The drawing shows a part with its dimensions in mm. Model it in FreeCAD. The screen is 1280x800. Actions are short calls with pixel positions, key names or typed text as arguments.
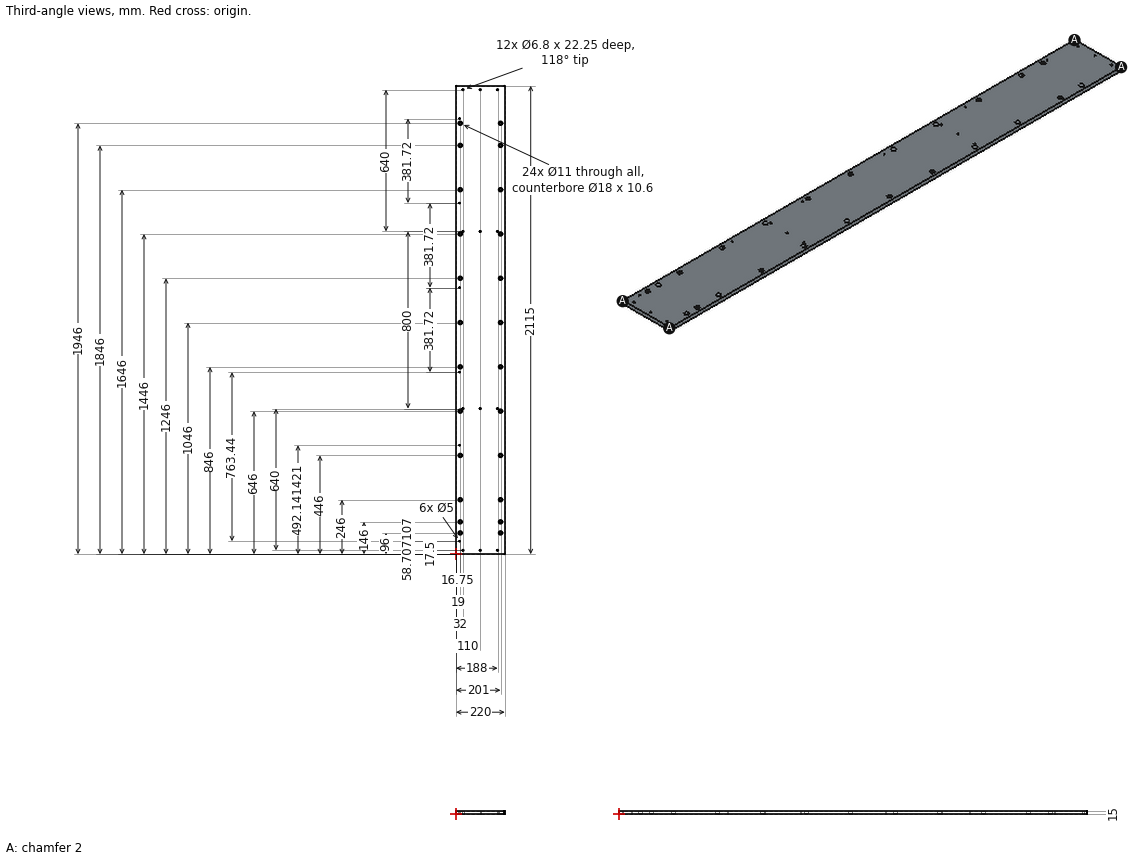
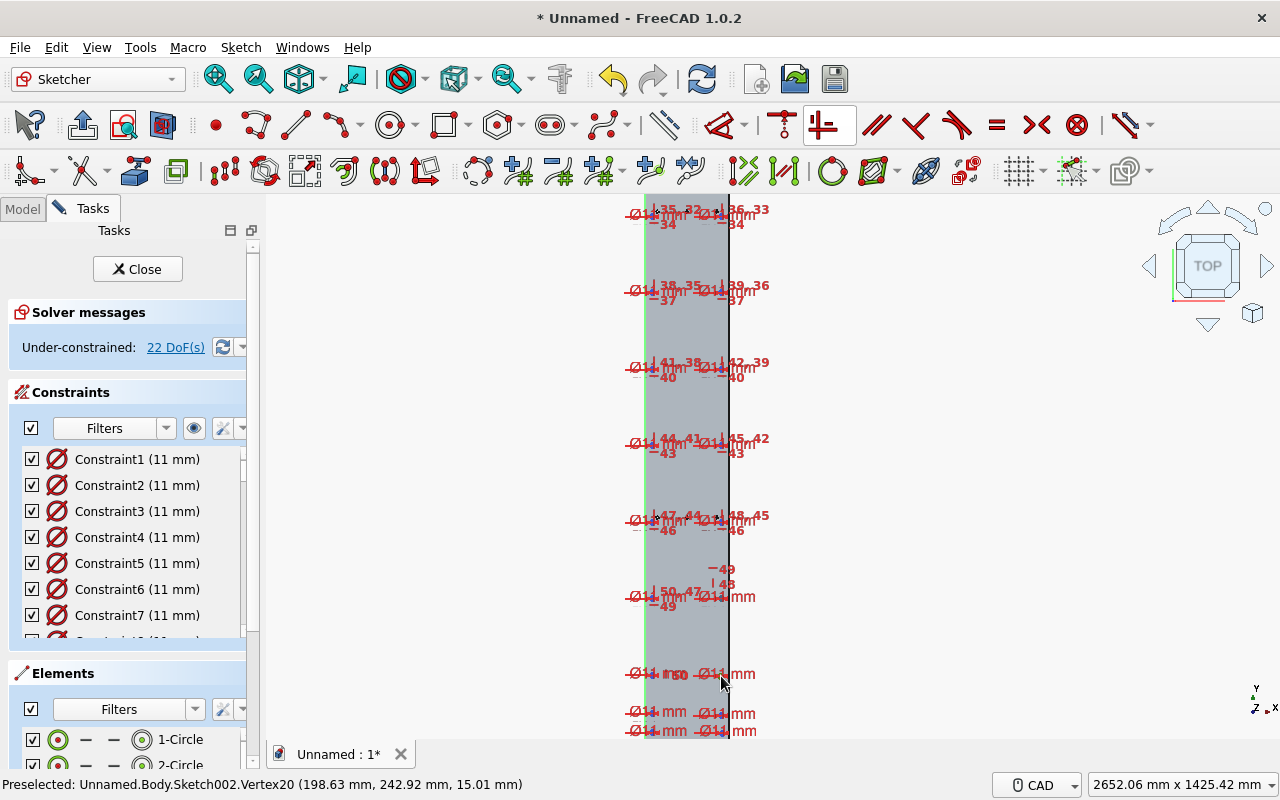
click(850, 126)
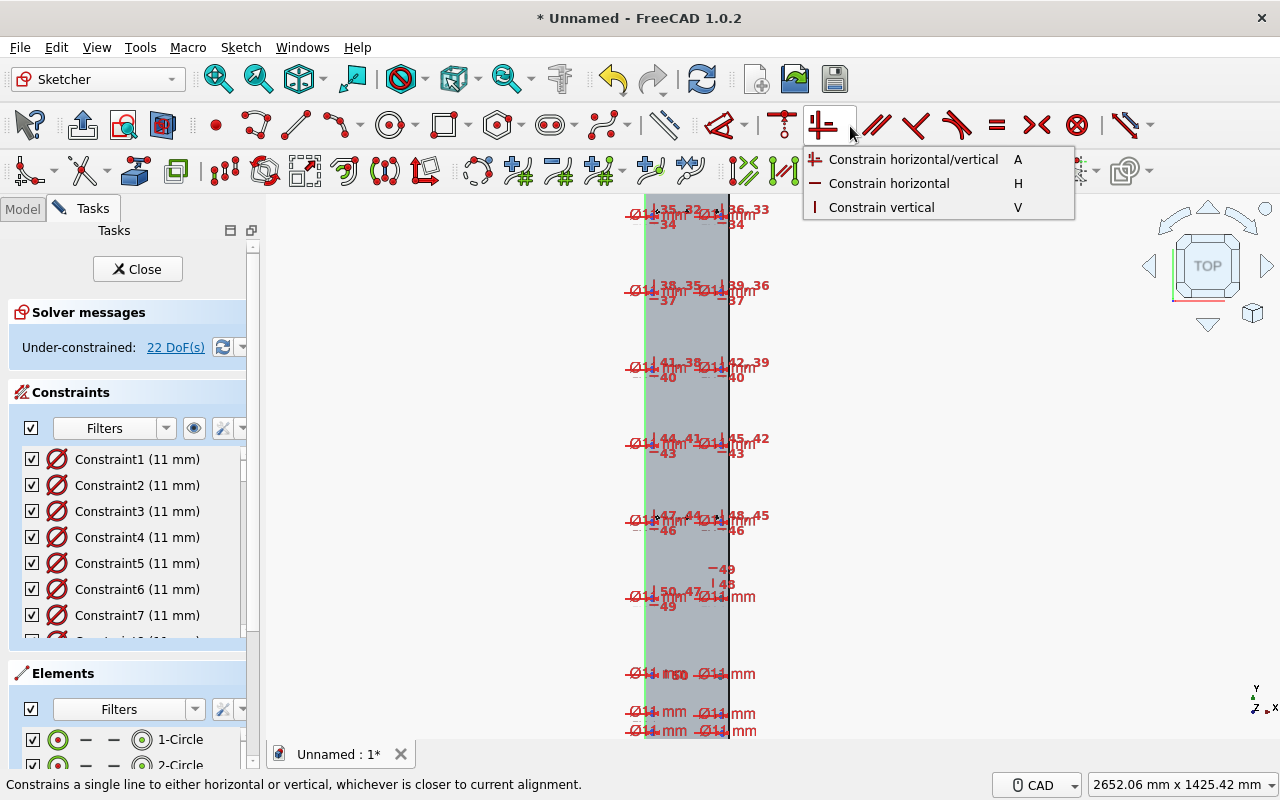
click(939, 207)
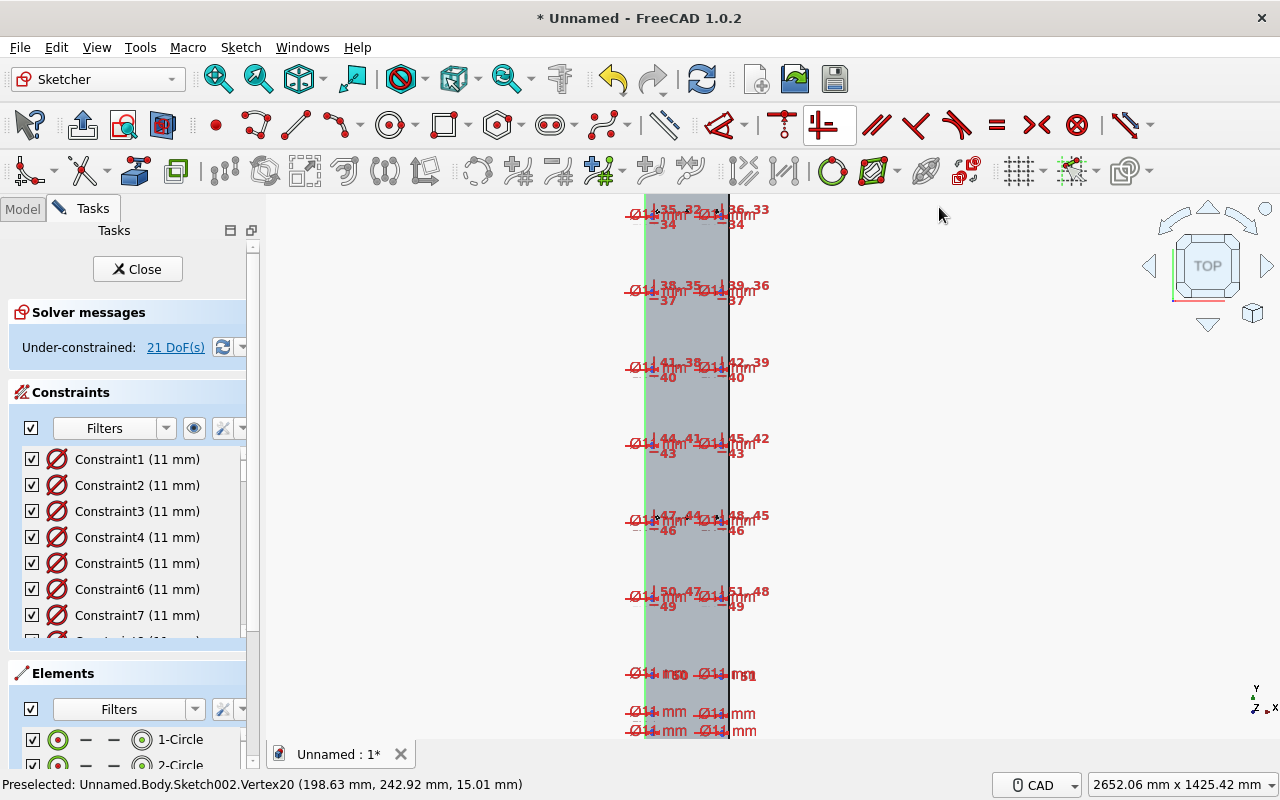
click(652, 675)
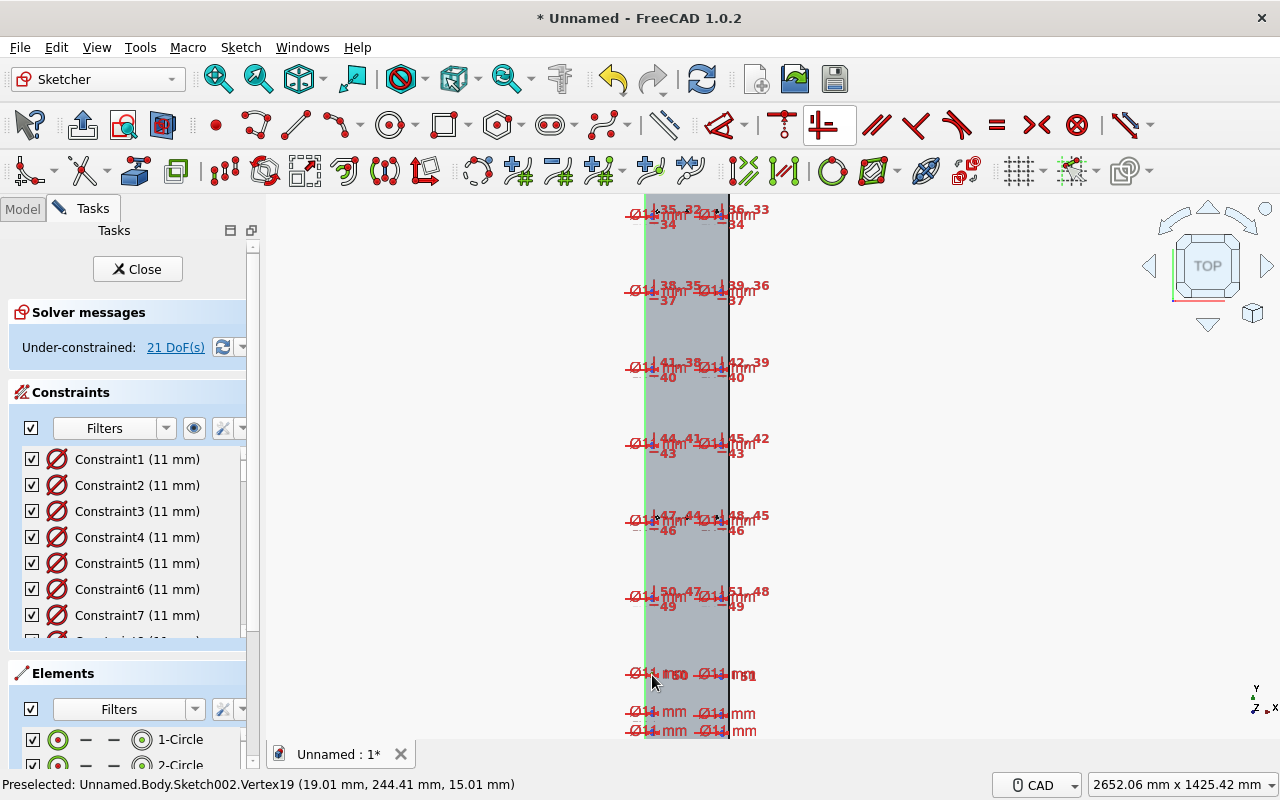
click(721, 676)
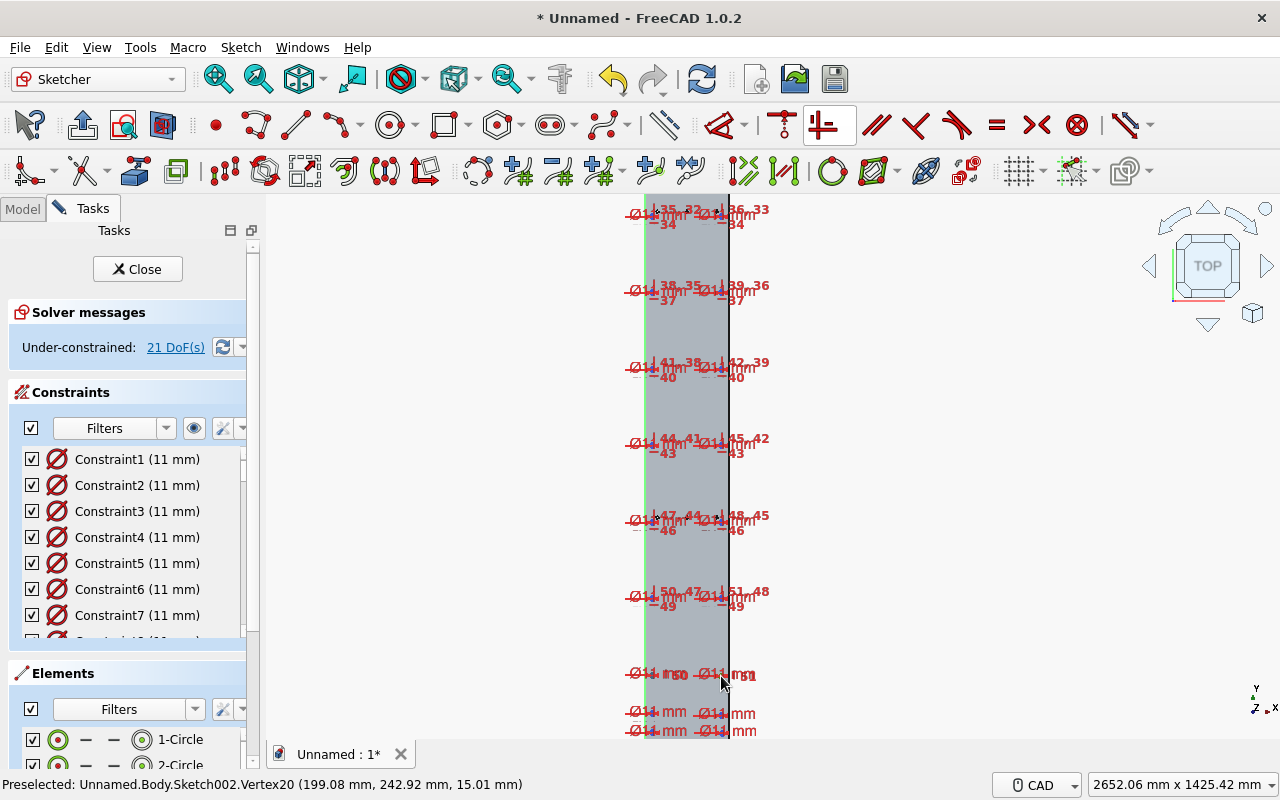
click(850, 126)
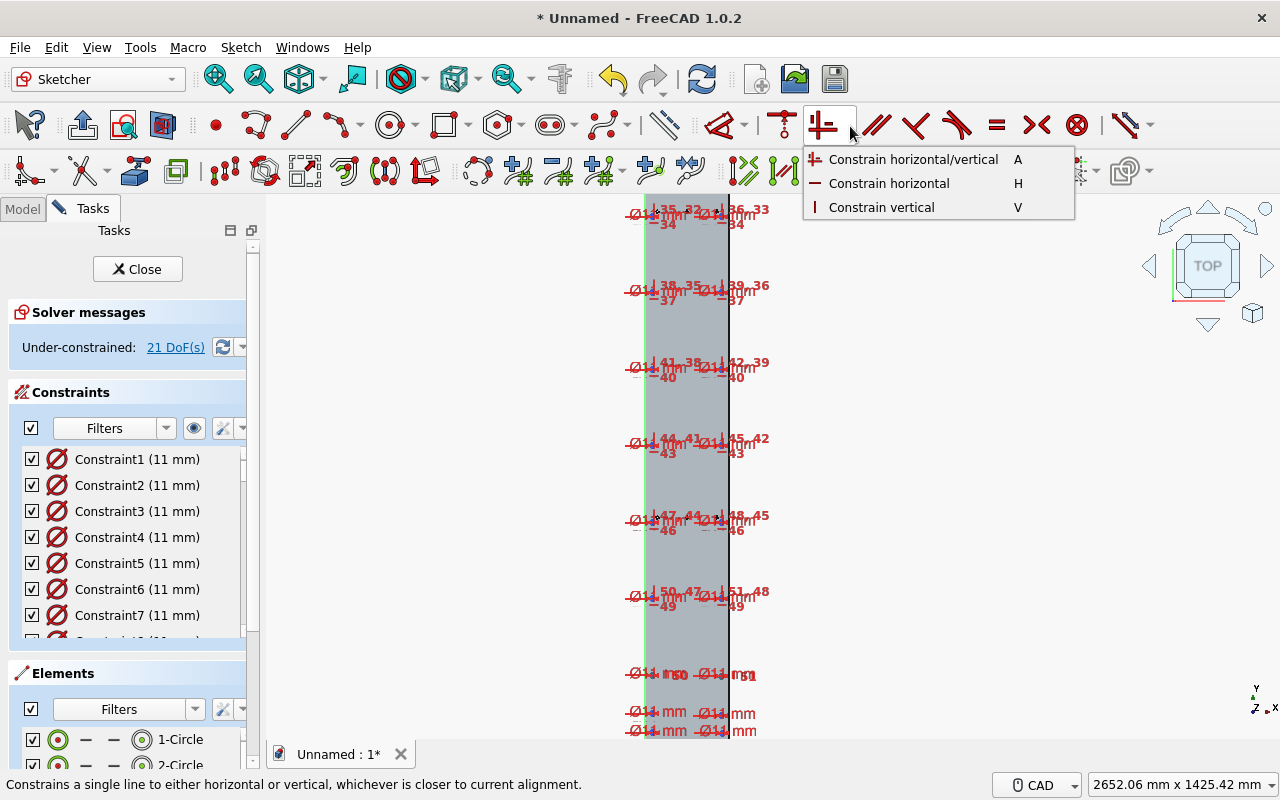
click(939, 183)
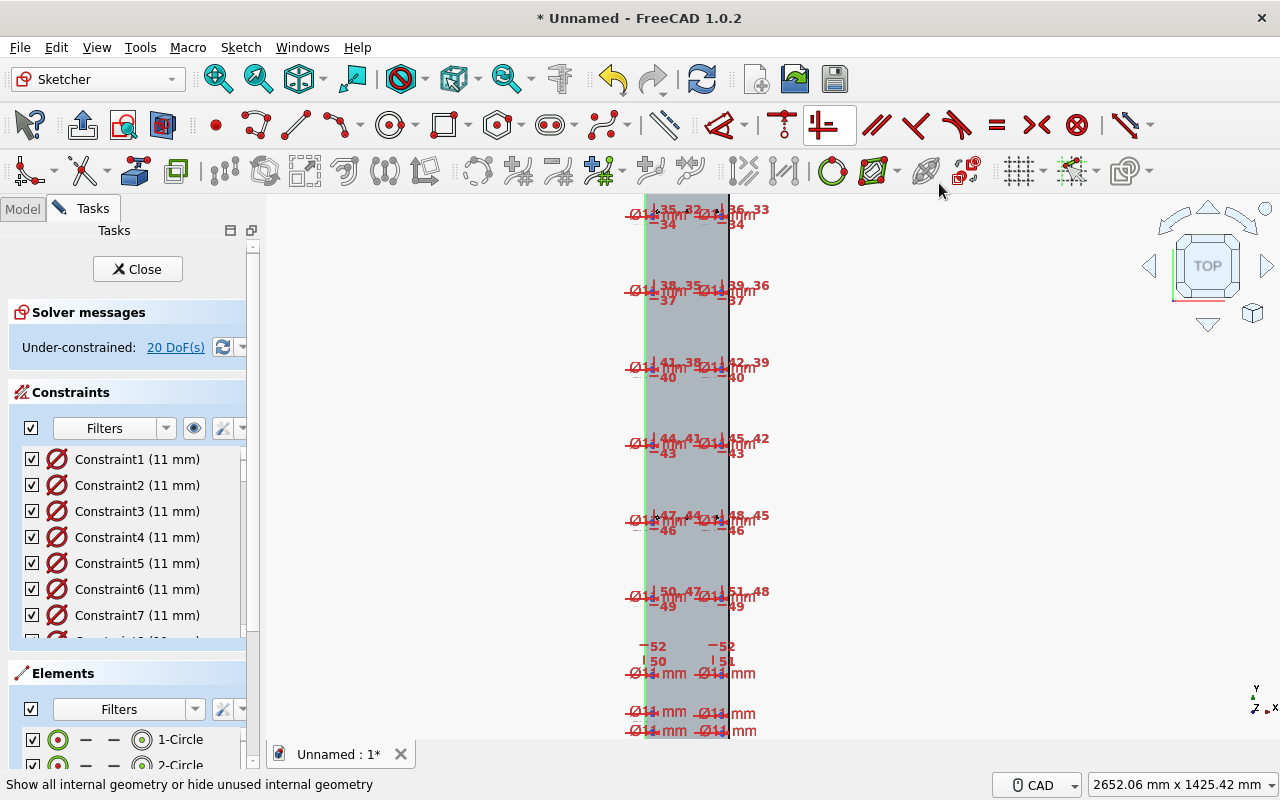
click(652, 675)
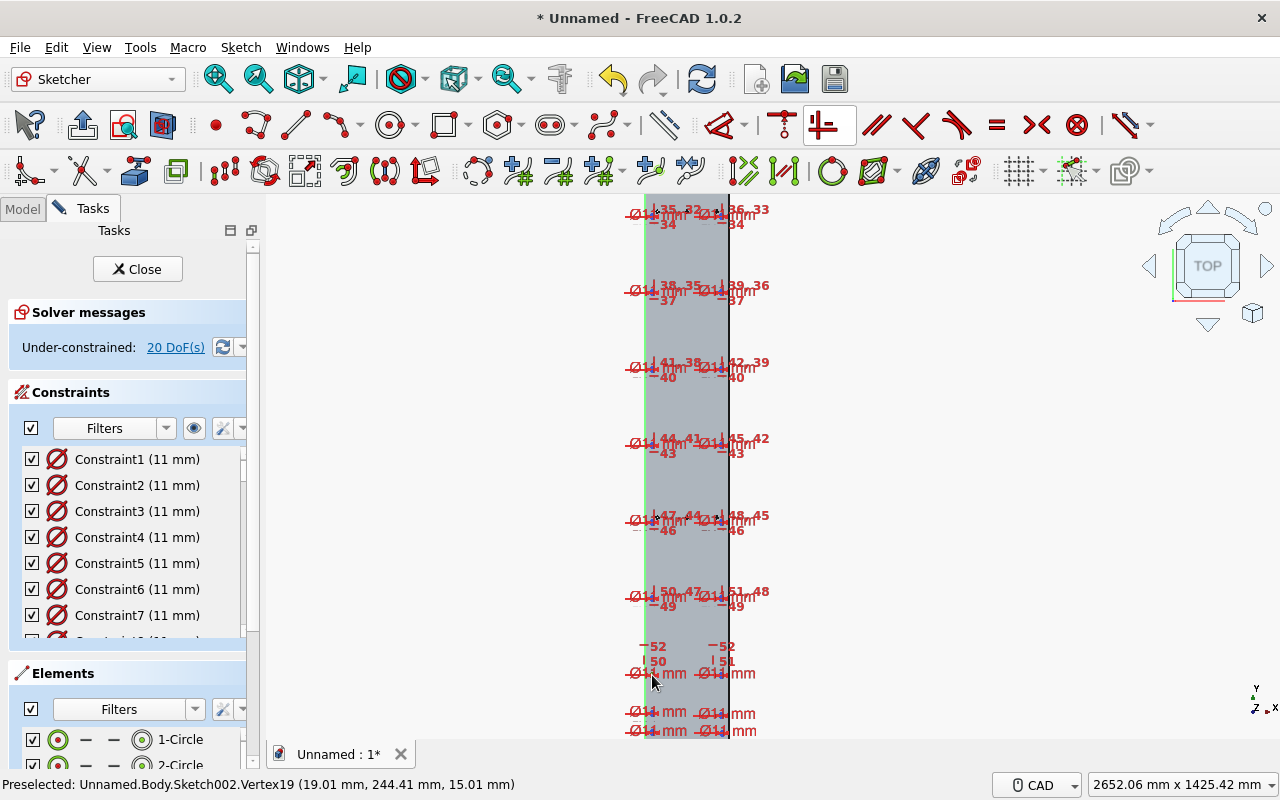
scroll(721, 524, down, 4)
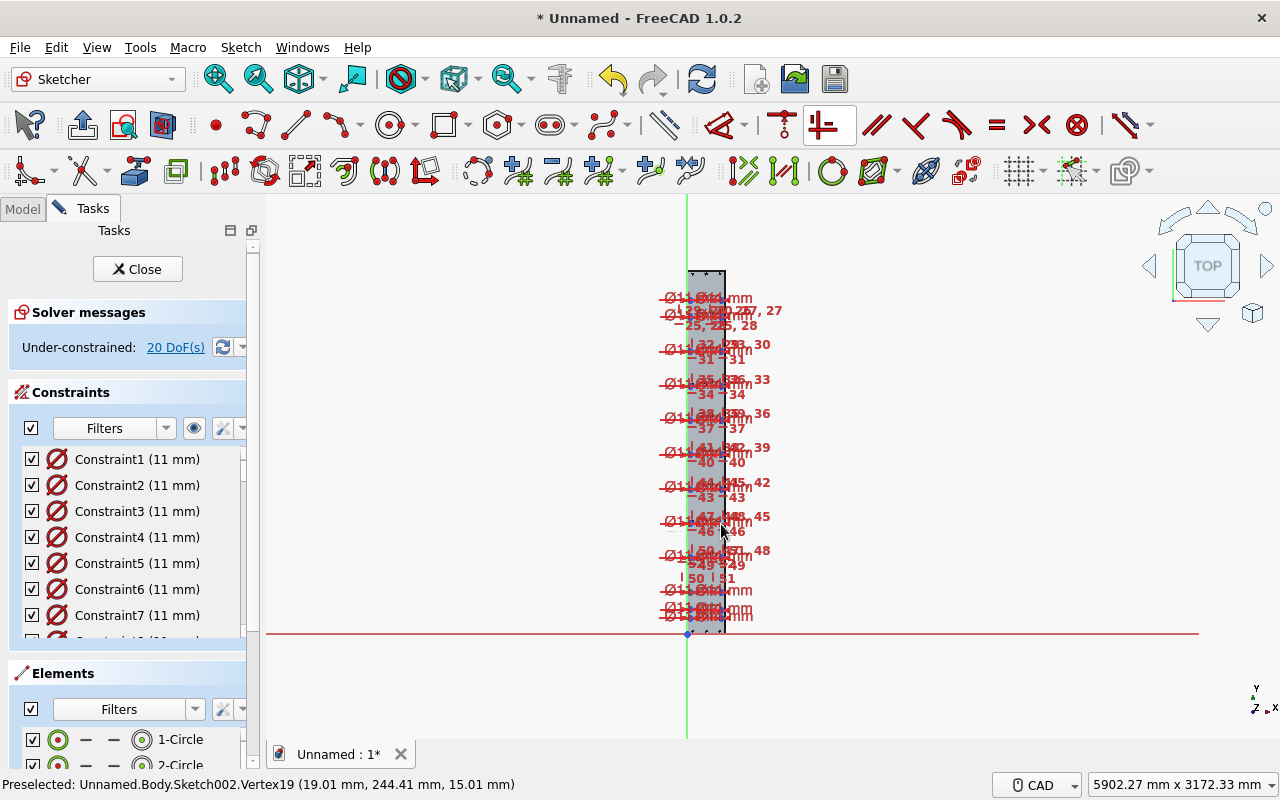
scroll(690, 610, up, 2)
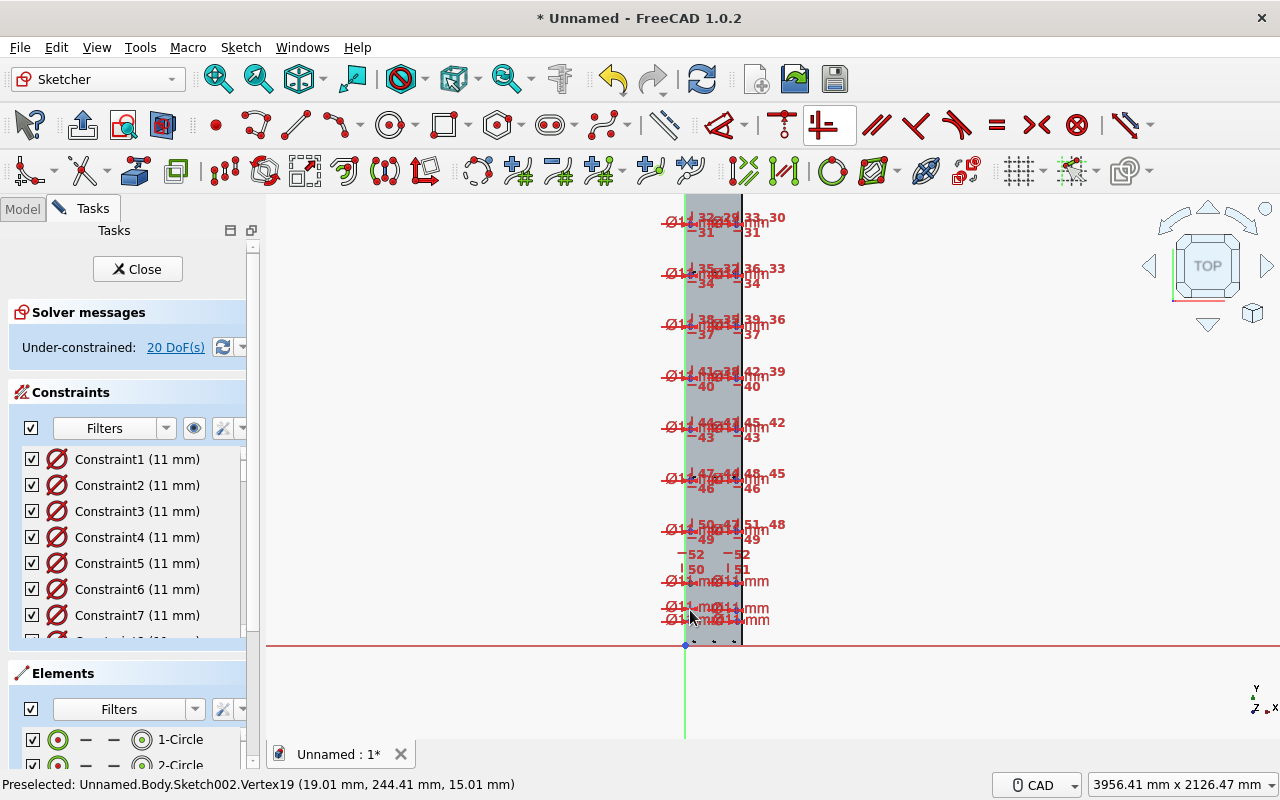
click(690, 609)